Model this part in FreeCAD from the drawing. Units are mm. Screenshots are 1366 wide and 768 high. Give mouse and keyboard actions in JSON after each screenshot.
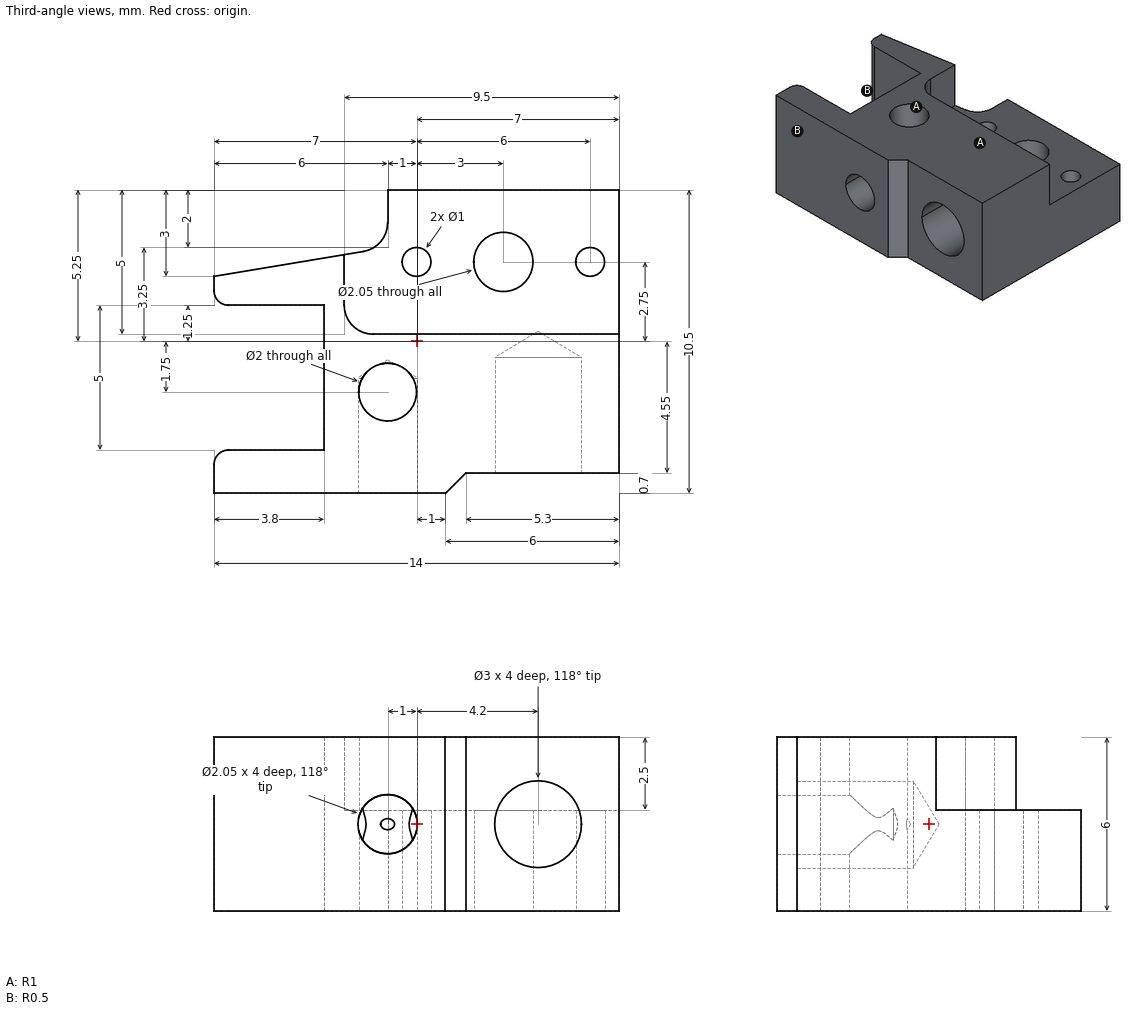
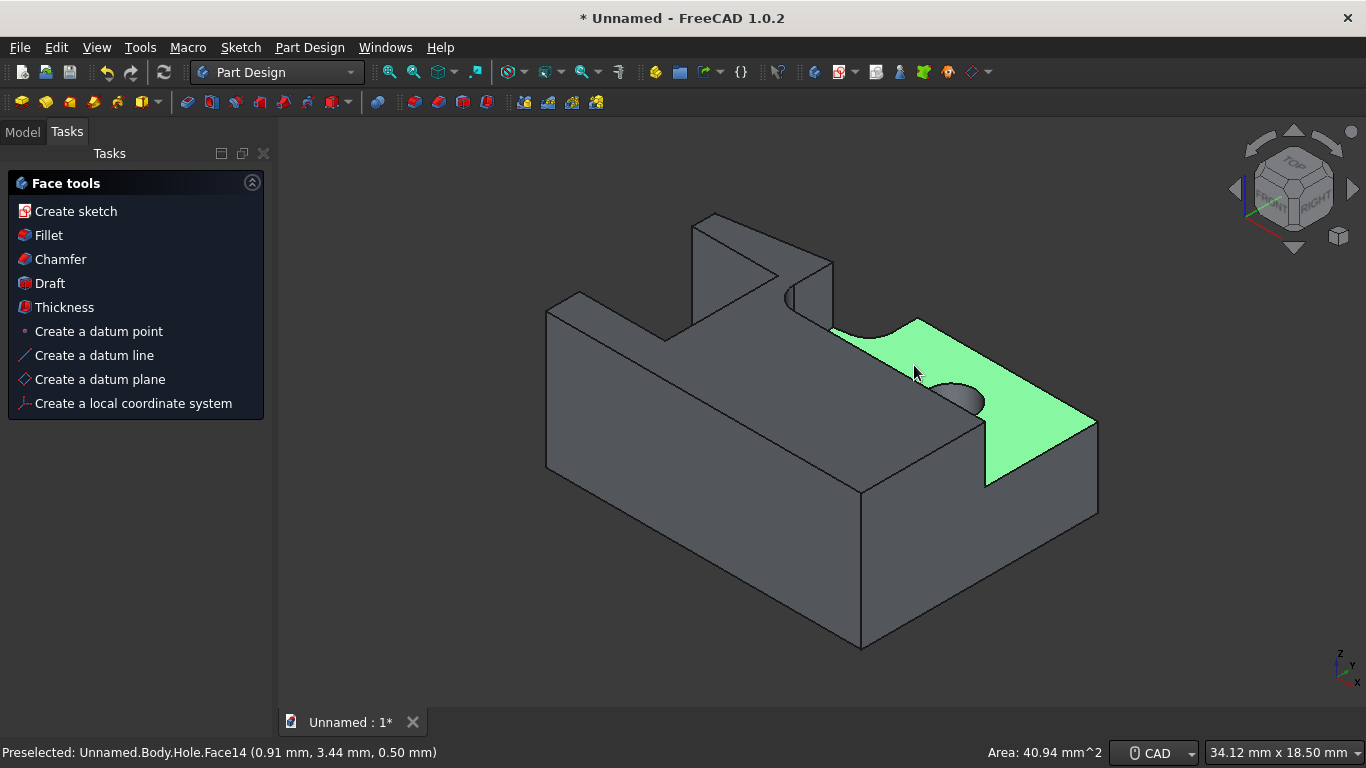
{"action": "left_click", "coordinate": [840, 72]}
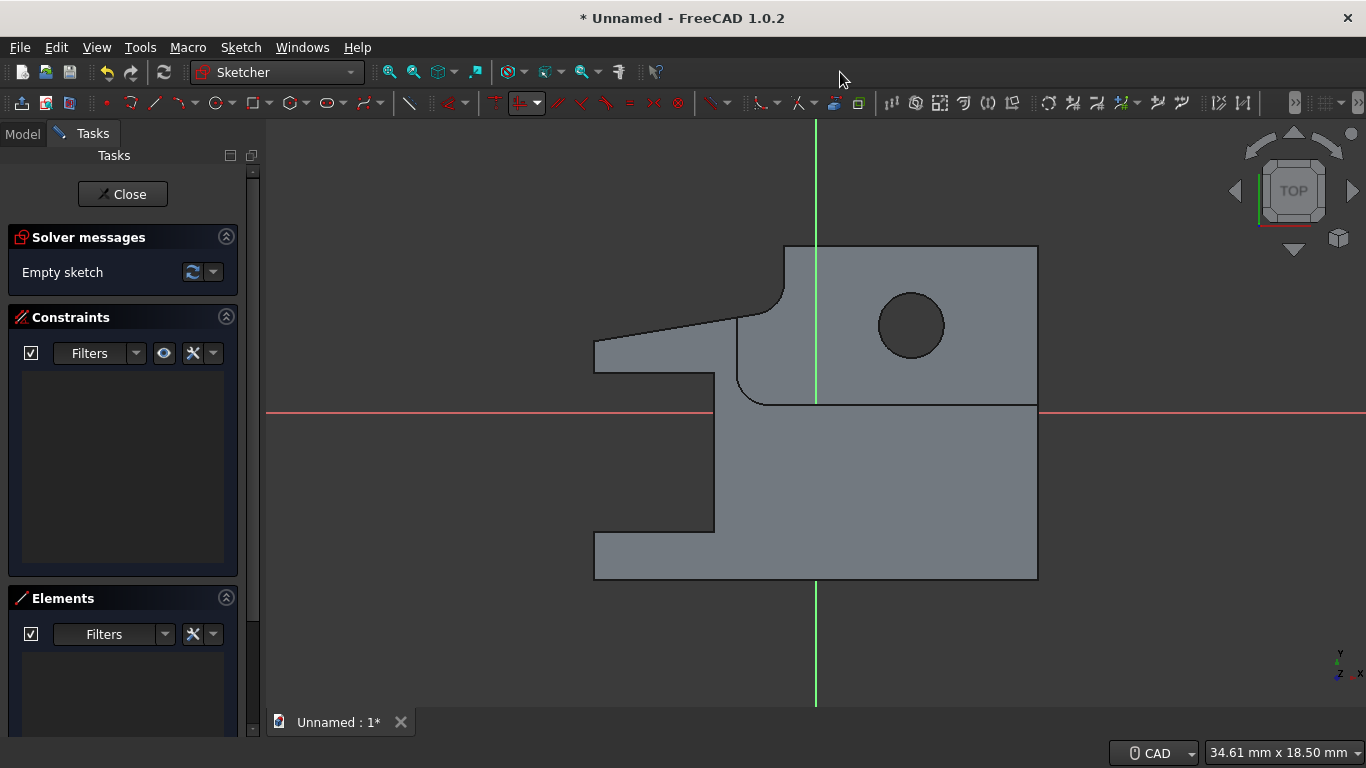
{"action": "scroll", "coordinate": [1007, 331], "scroll_direction": "up", "scroll_amount": 5}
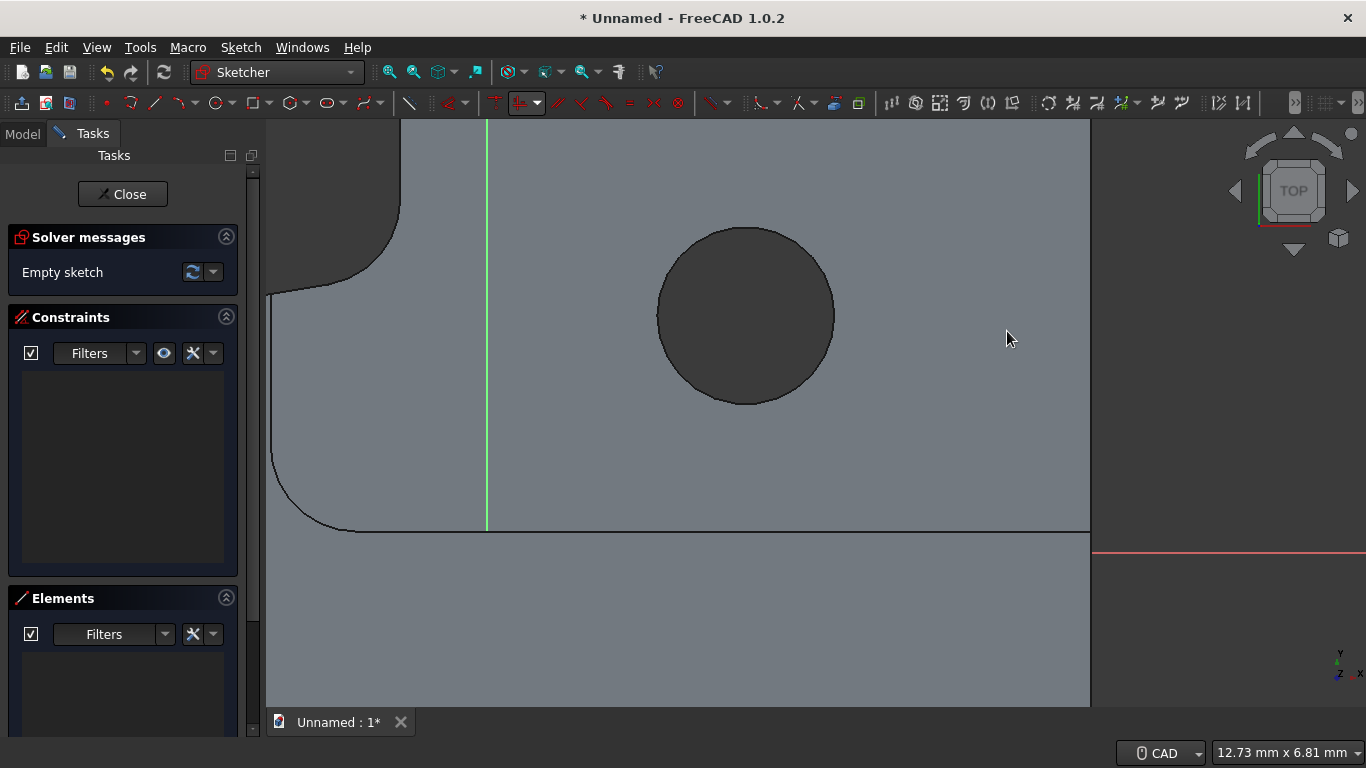
{"action": "left_click", "coordinate": [216, 104]}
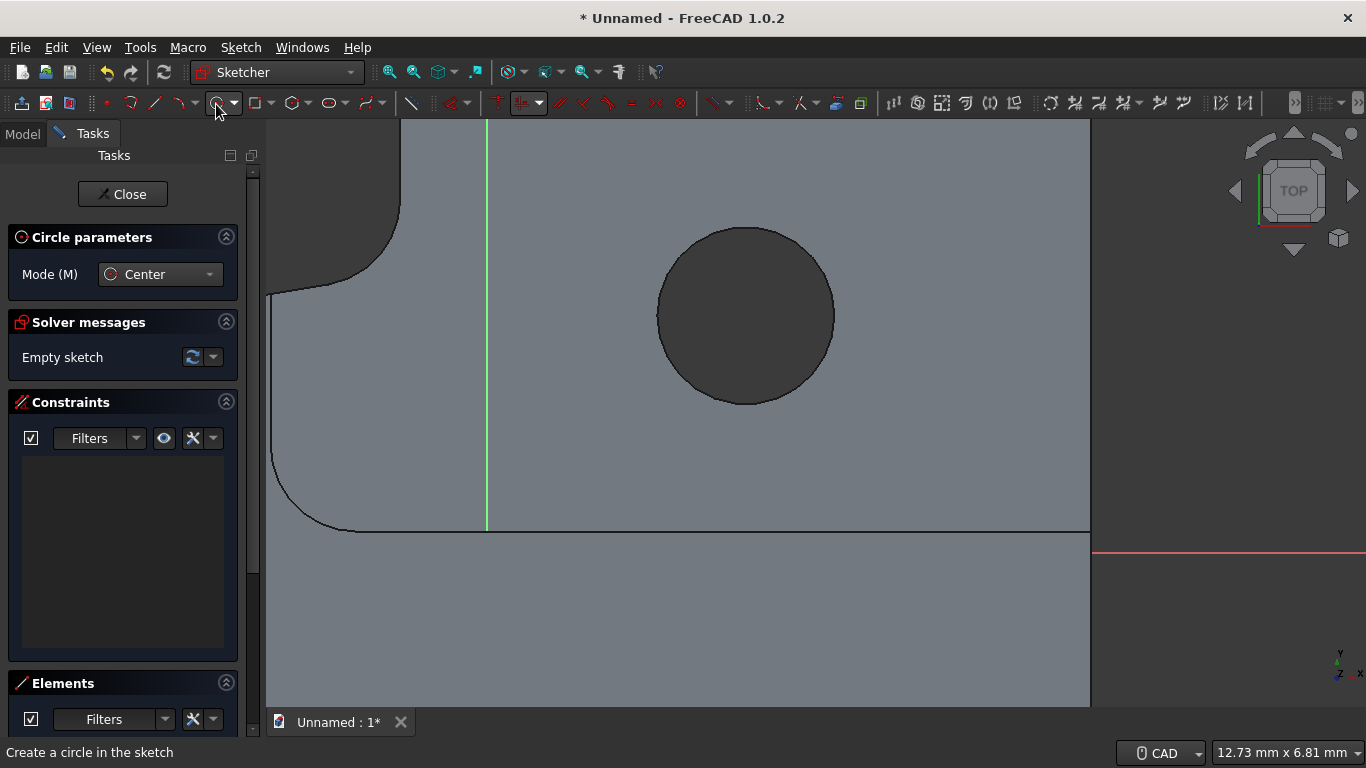
{"action": "left_click", "coordinate": [487, 316]}
{"action": "left_click", "coordinate": [517, 285]}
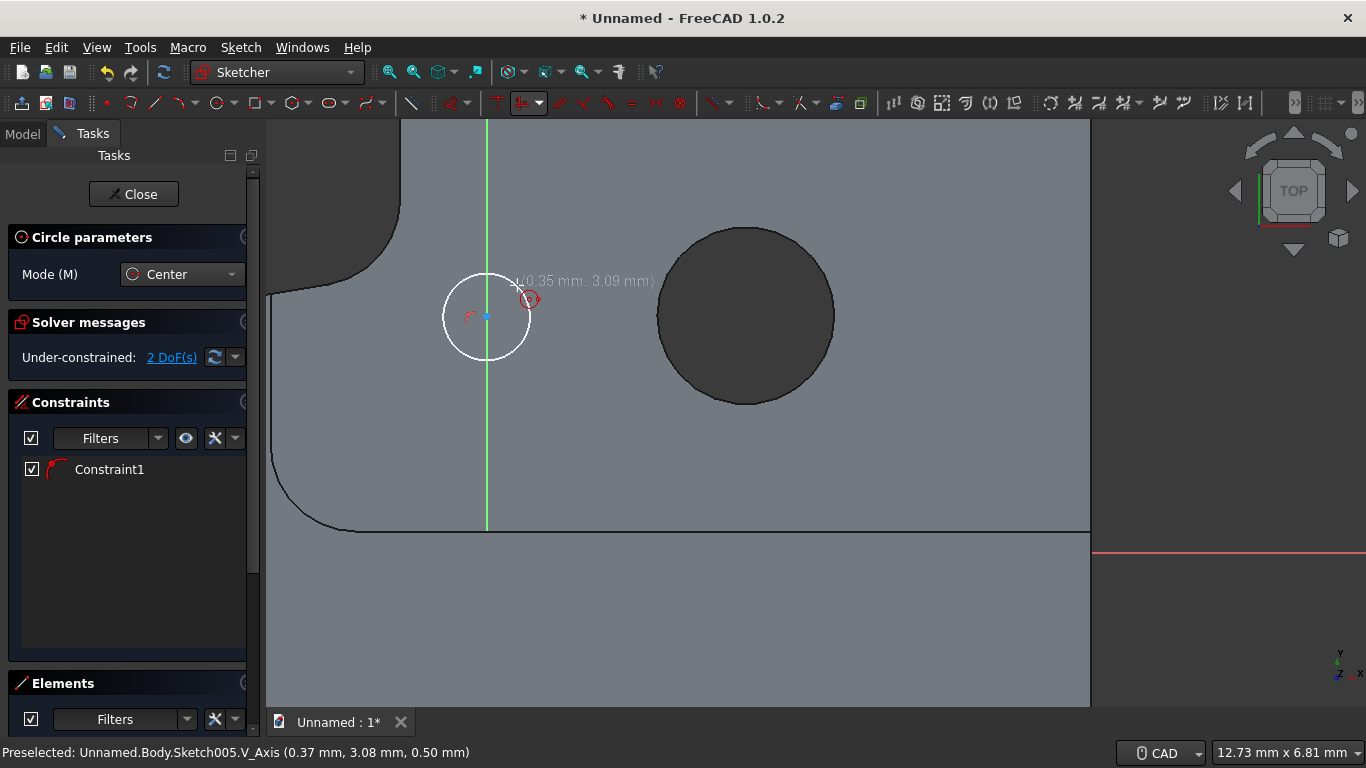
{"action": "left_click", "coordinate": [1005, 316]}
{"action": "left_click", "coordinate": [1036, 285]}
{"action": "key", "text": "Escape"}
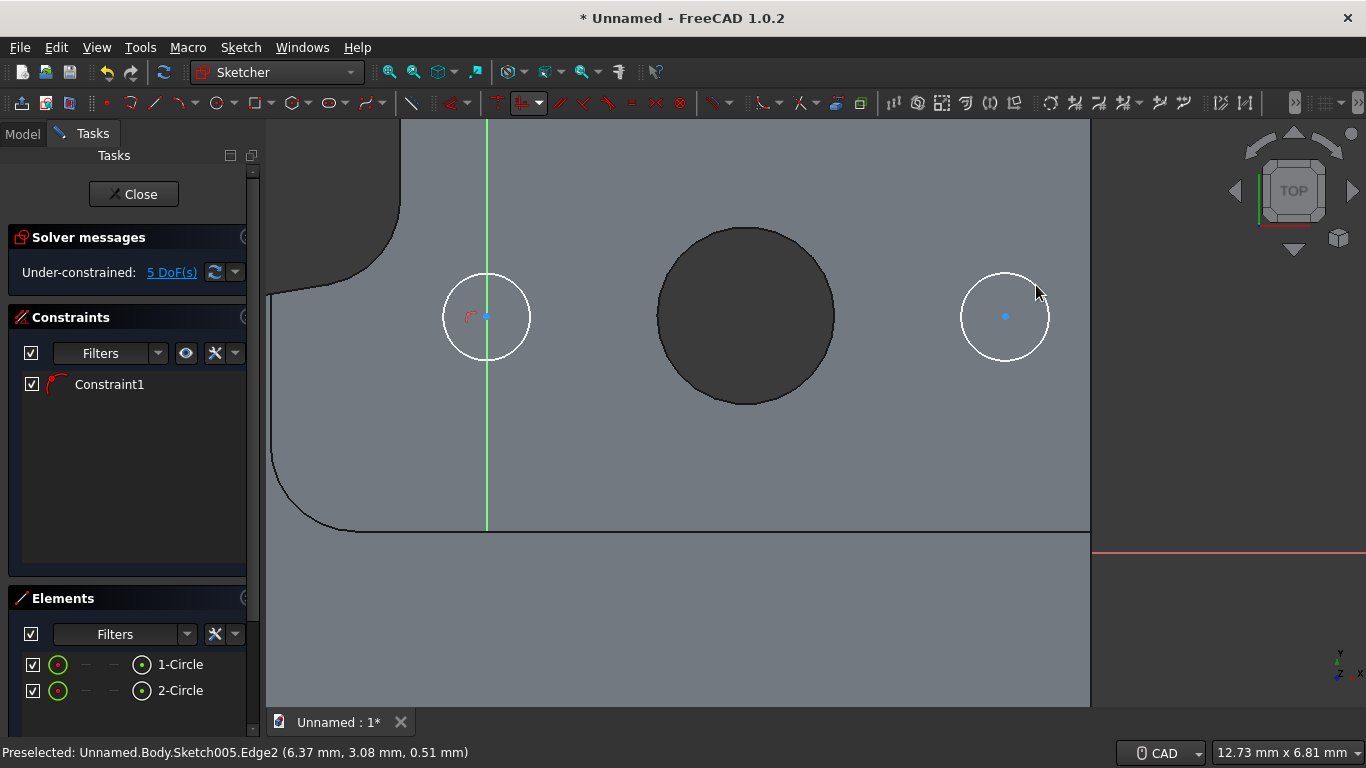
{"action": "left_click", "coordinate": [517, 286]}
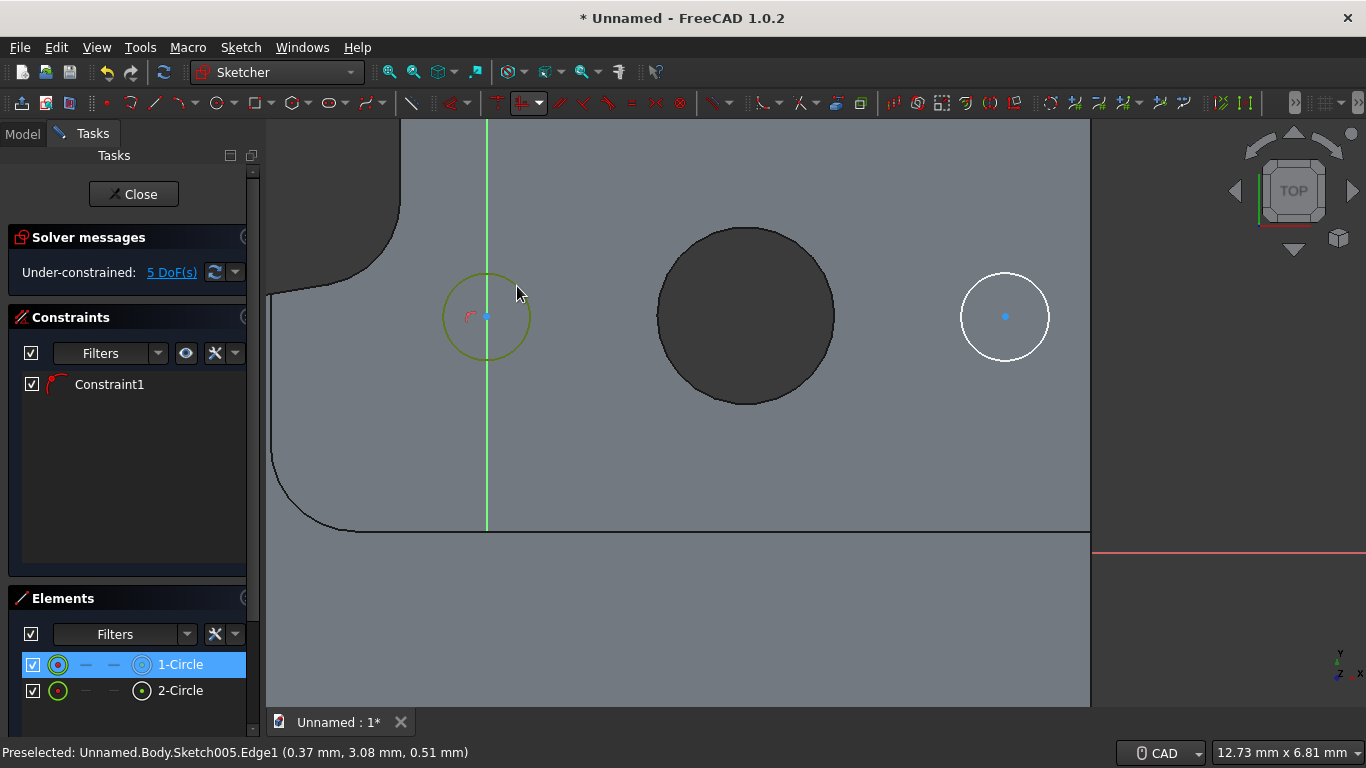
{"action": "left_click", "coordinate": [1036, 286]}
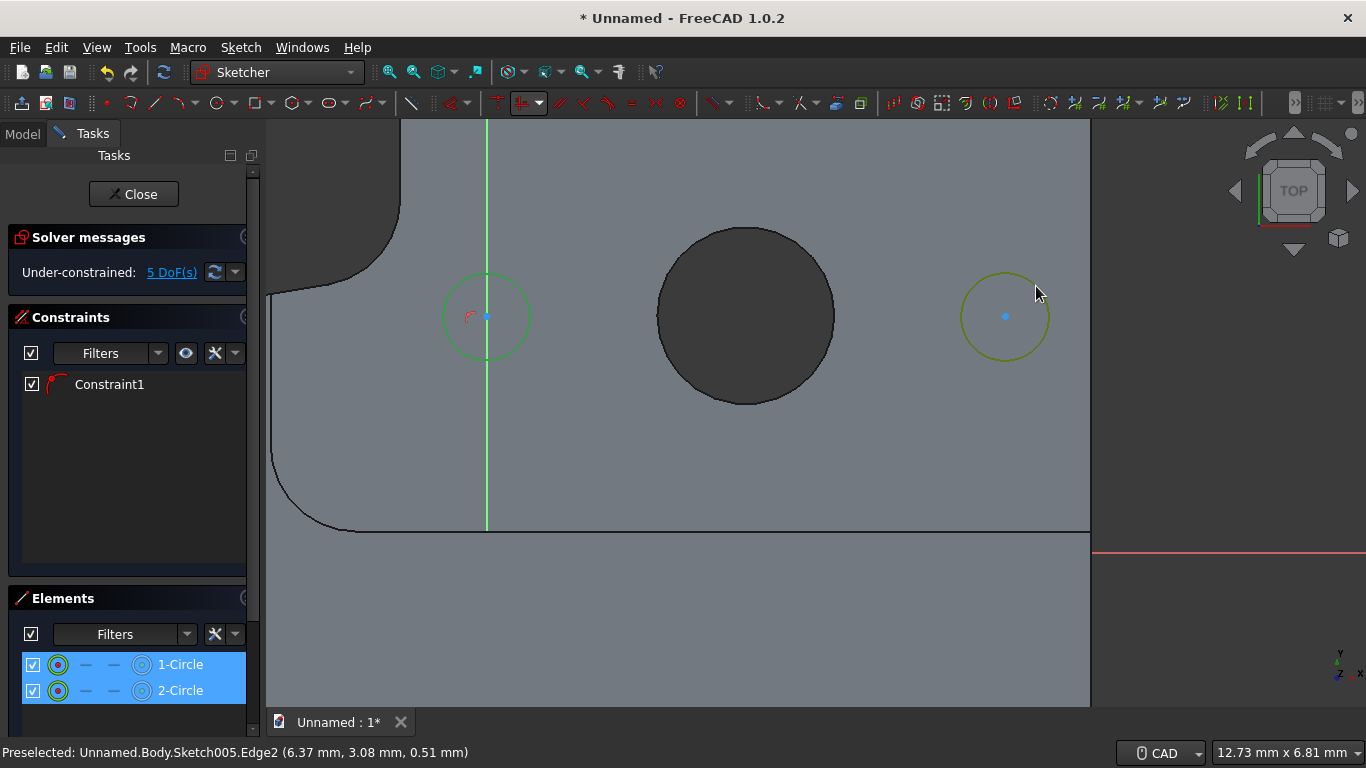
{"action": "left_click", "coordinate": [632, 104]}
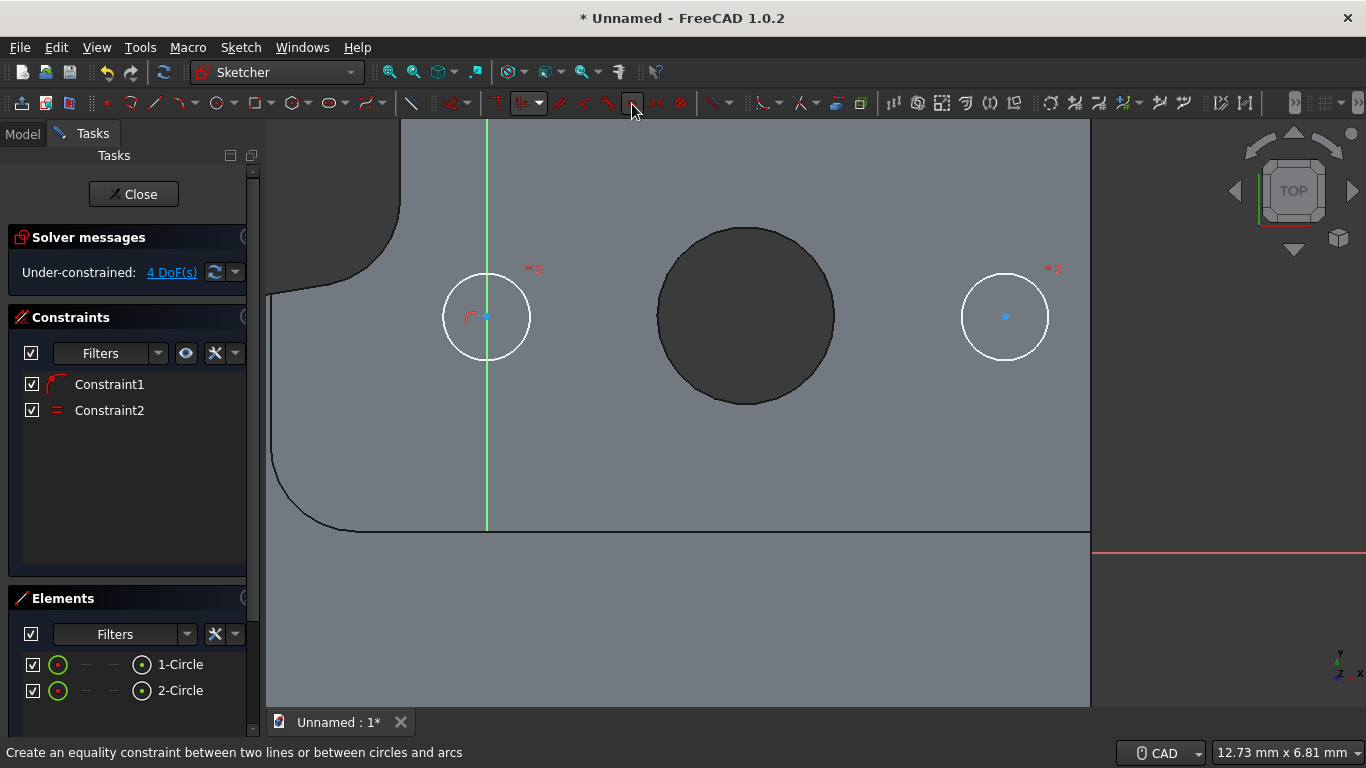
{"action": "left_click", "coordinate": [450, 104]}